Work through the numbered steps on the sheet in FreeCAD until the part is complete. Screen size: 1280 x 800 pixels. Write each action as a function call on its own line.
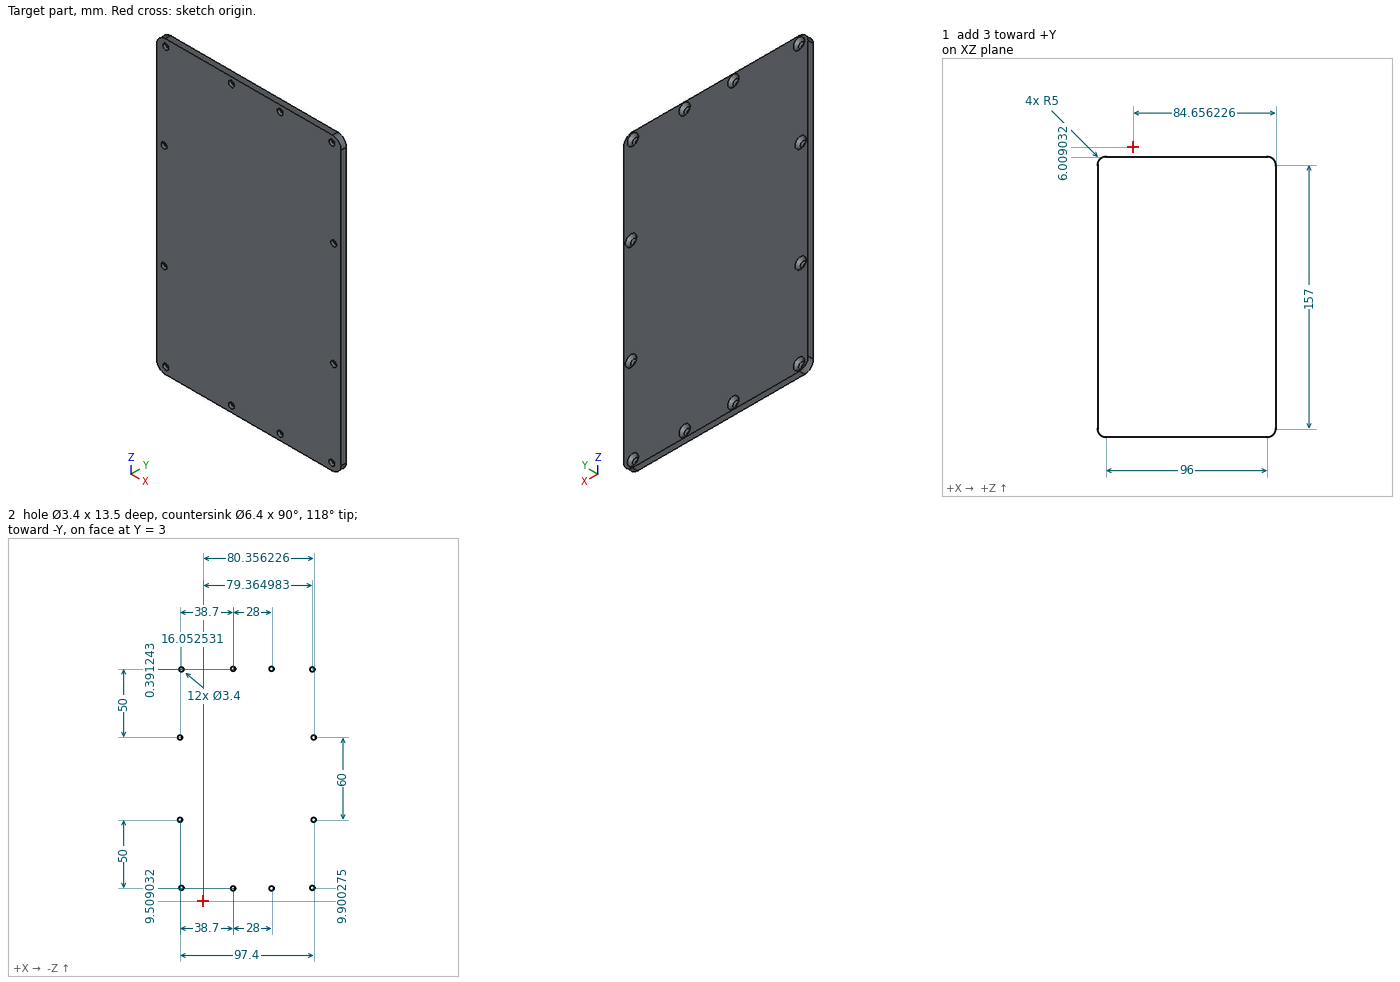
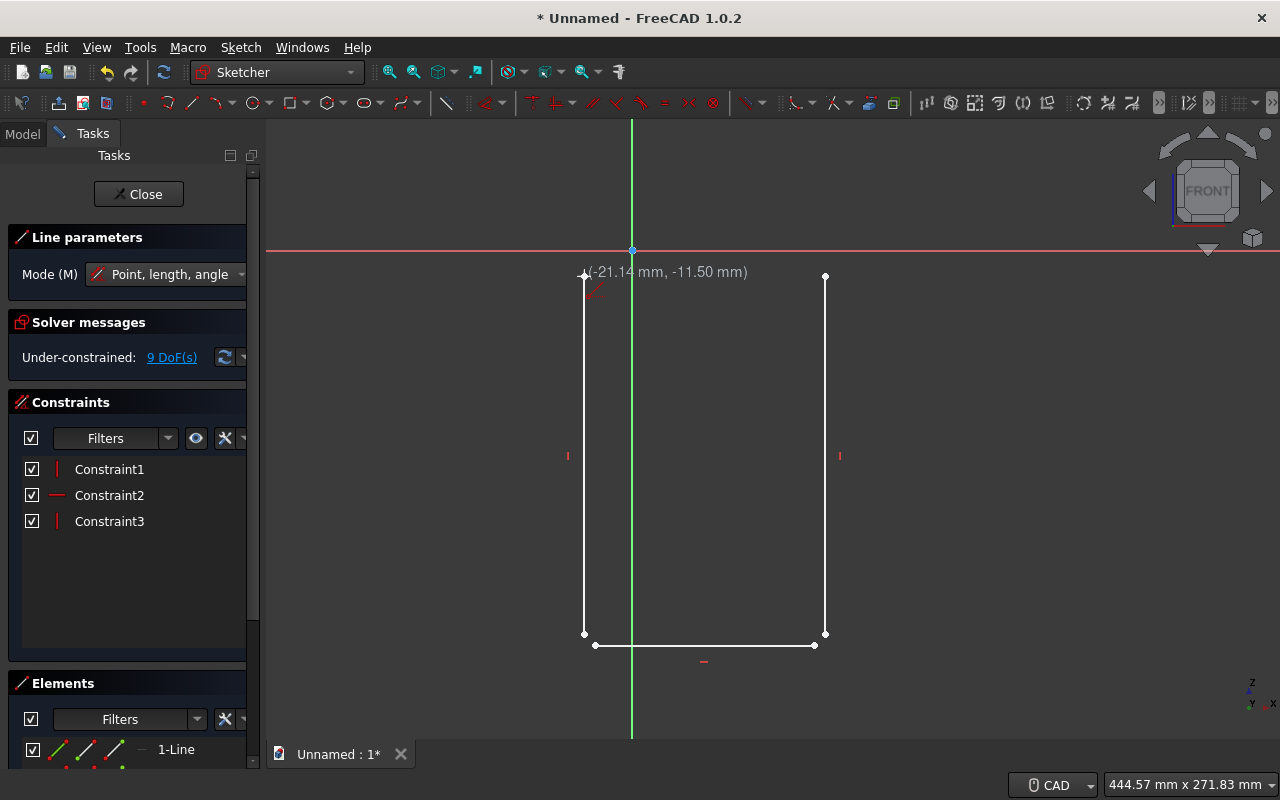
click(595, 264)
click(814, 264)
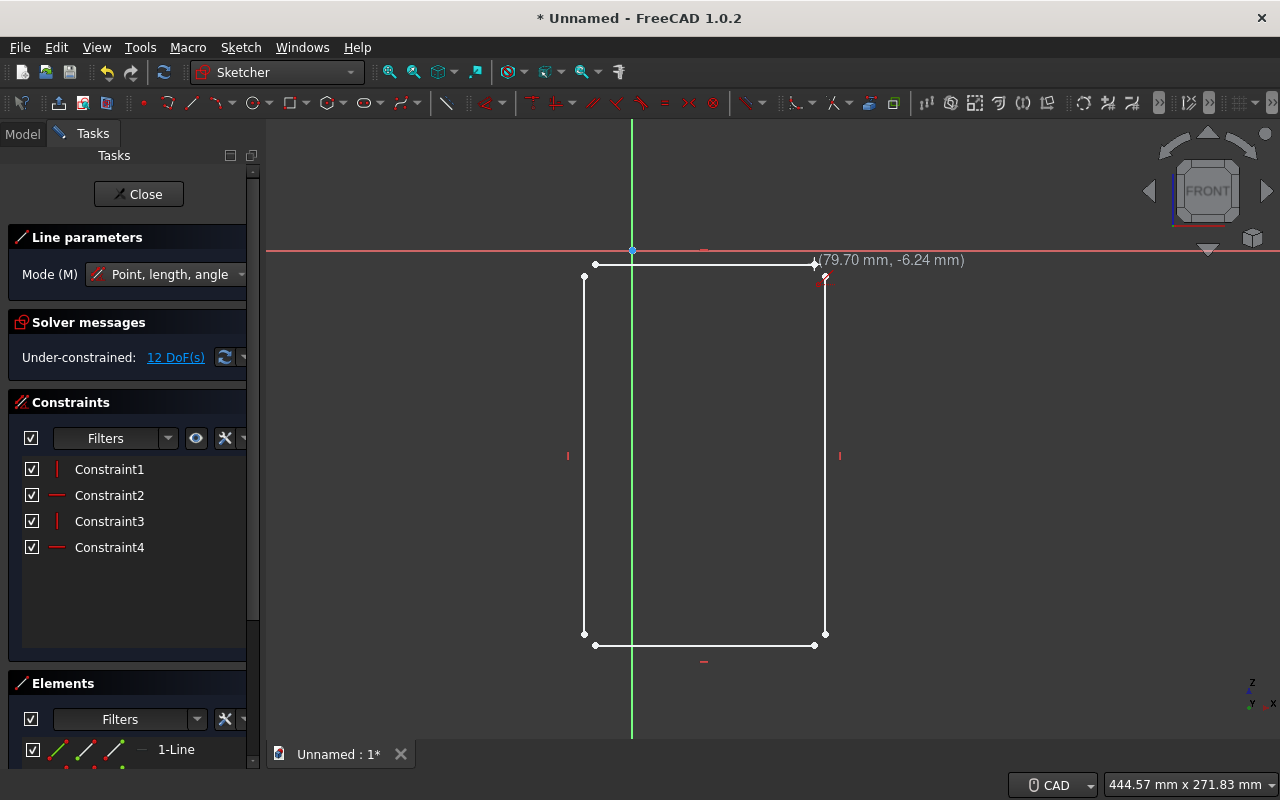
click(216, 104)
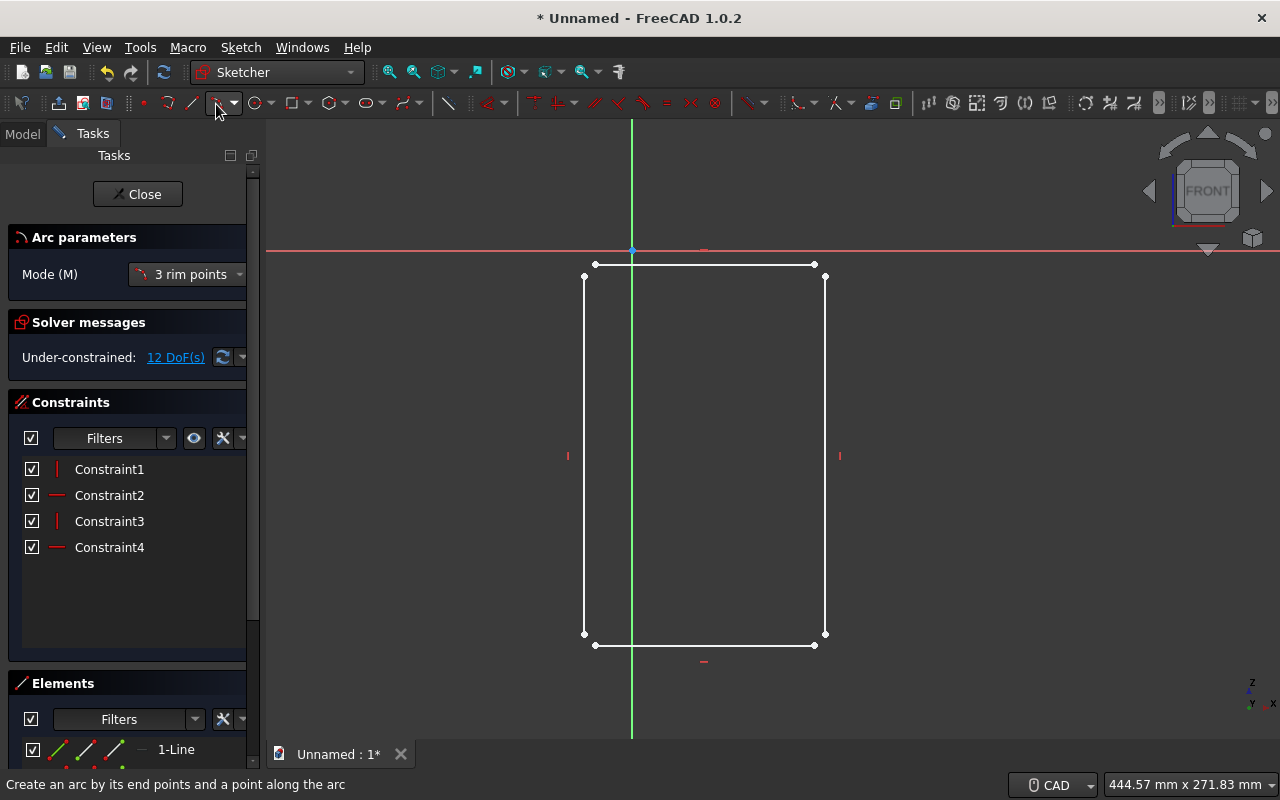
click(825, 635)
click(814, 646)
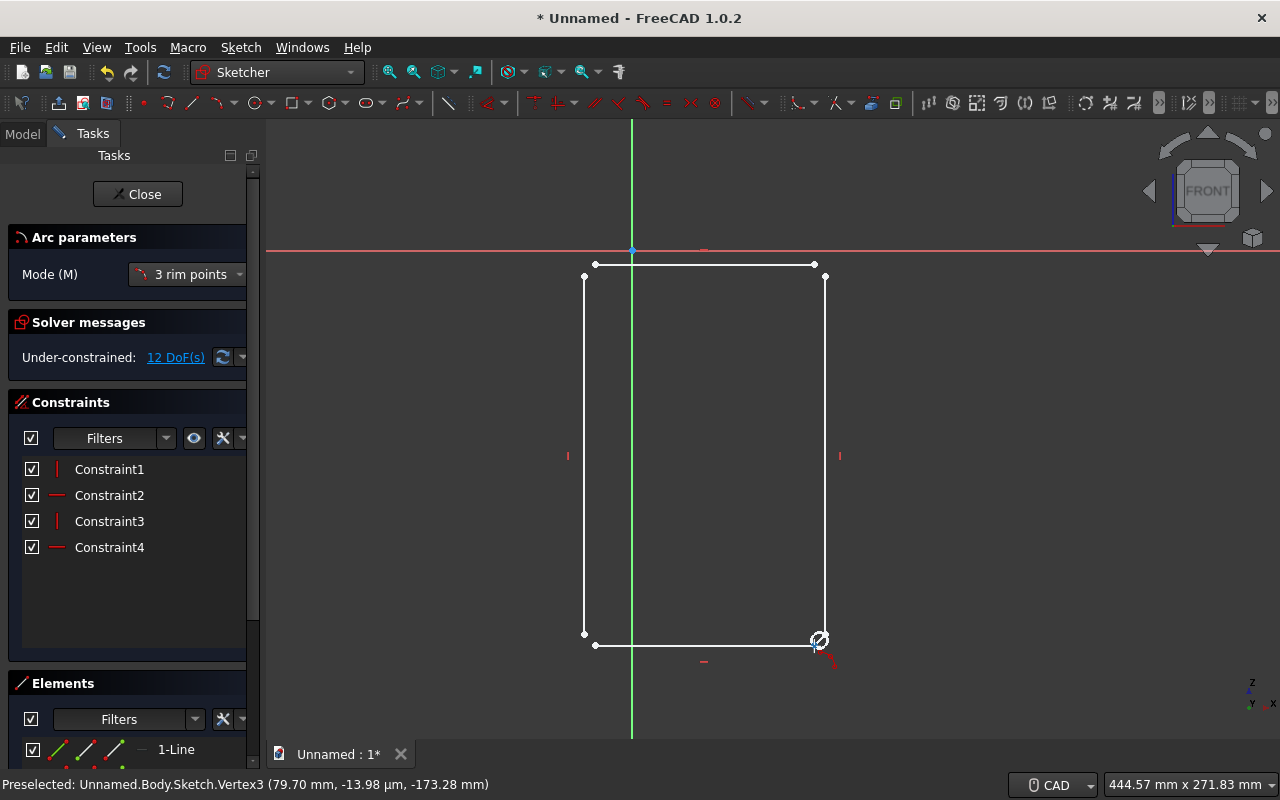
scroll(822, 642, up, 8)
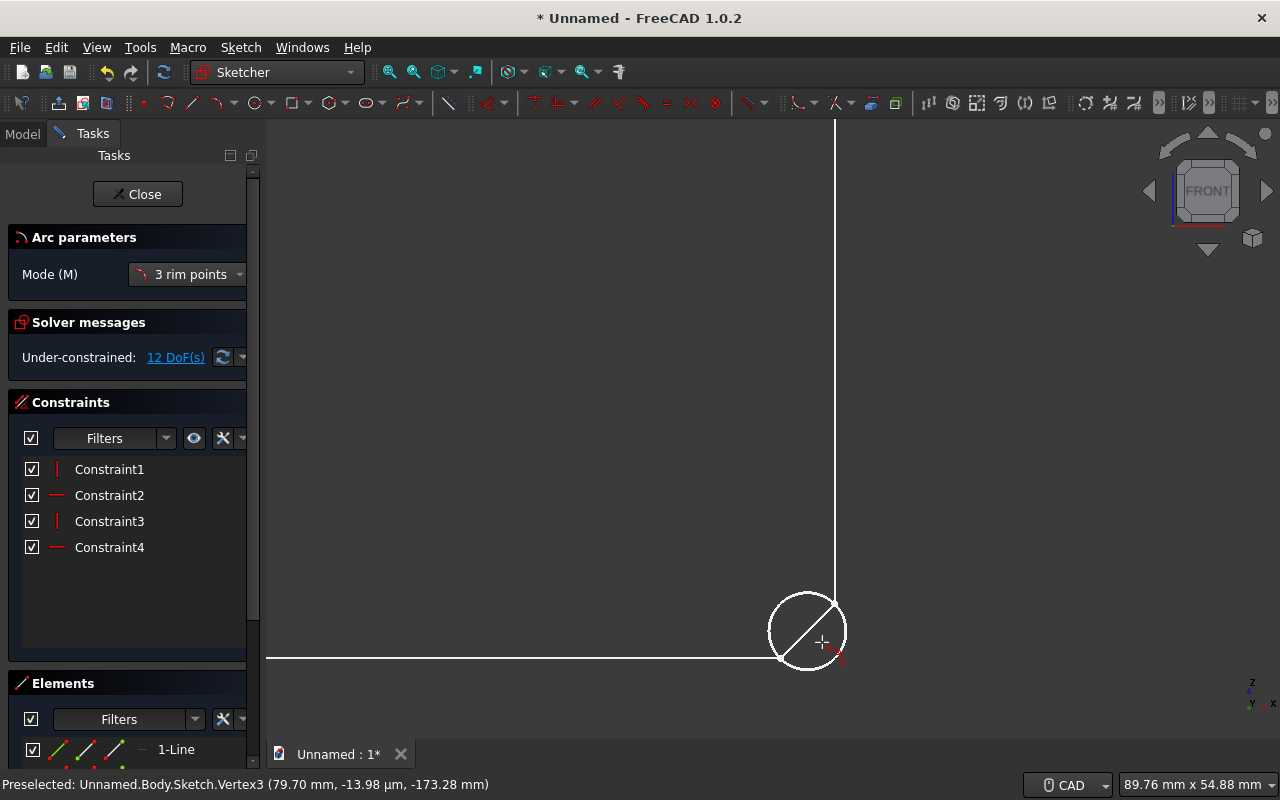
click(820, 639)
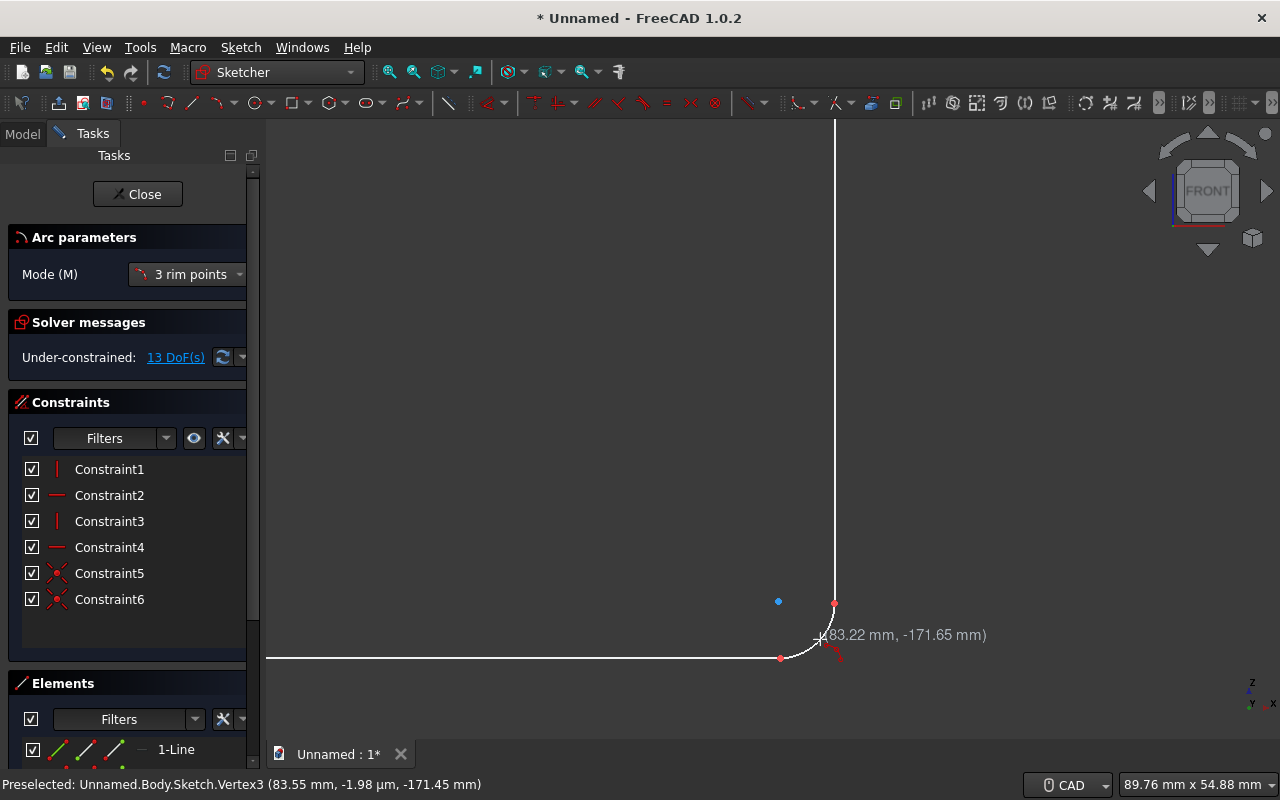
scroll(823, 619, down, 8)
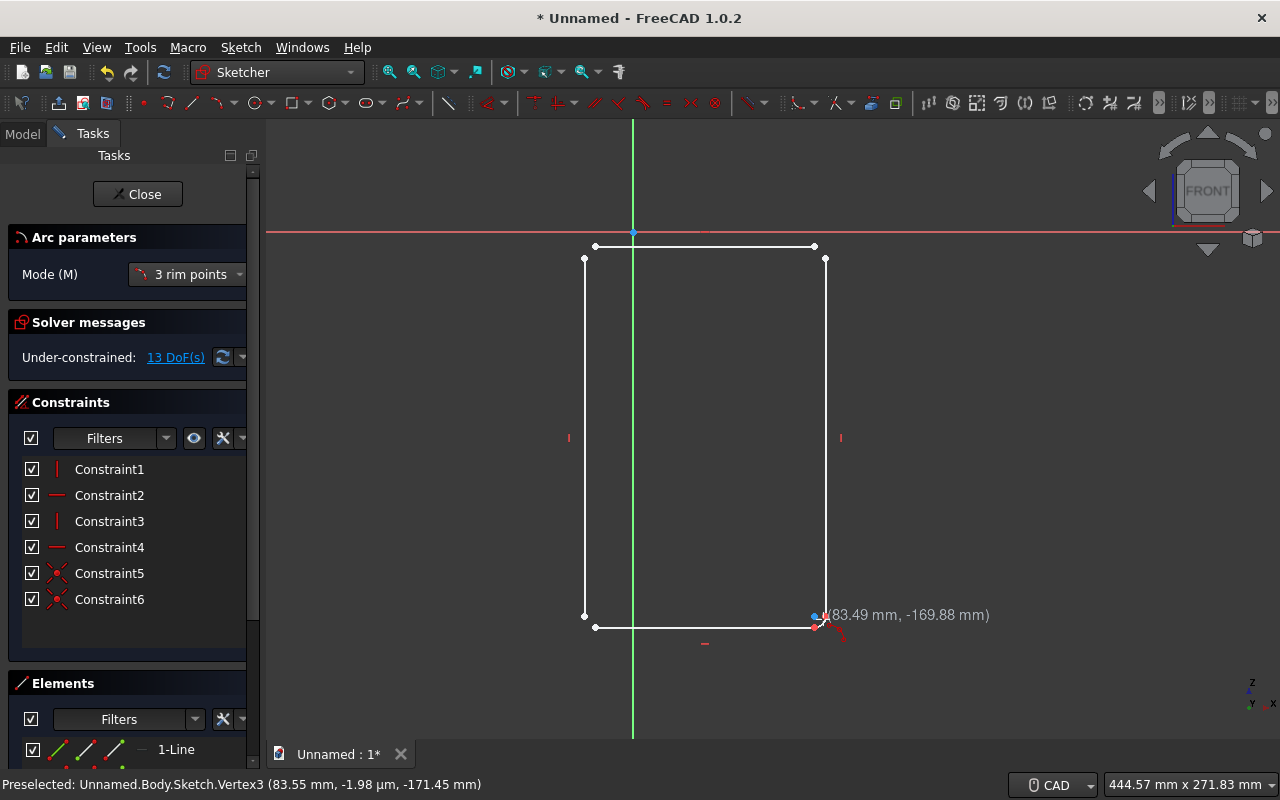
click(596, 628)
click(585, 617)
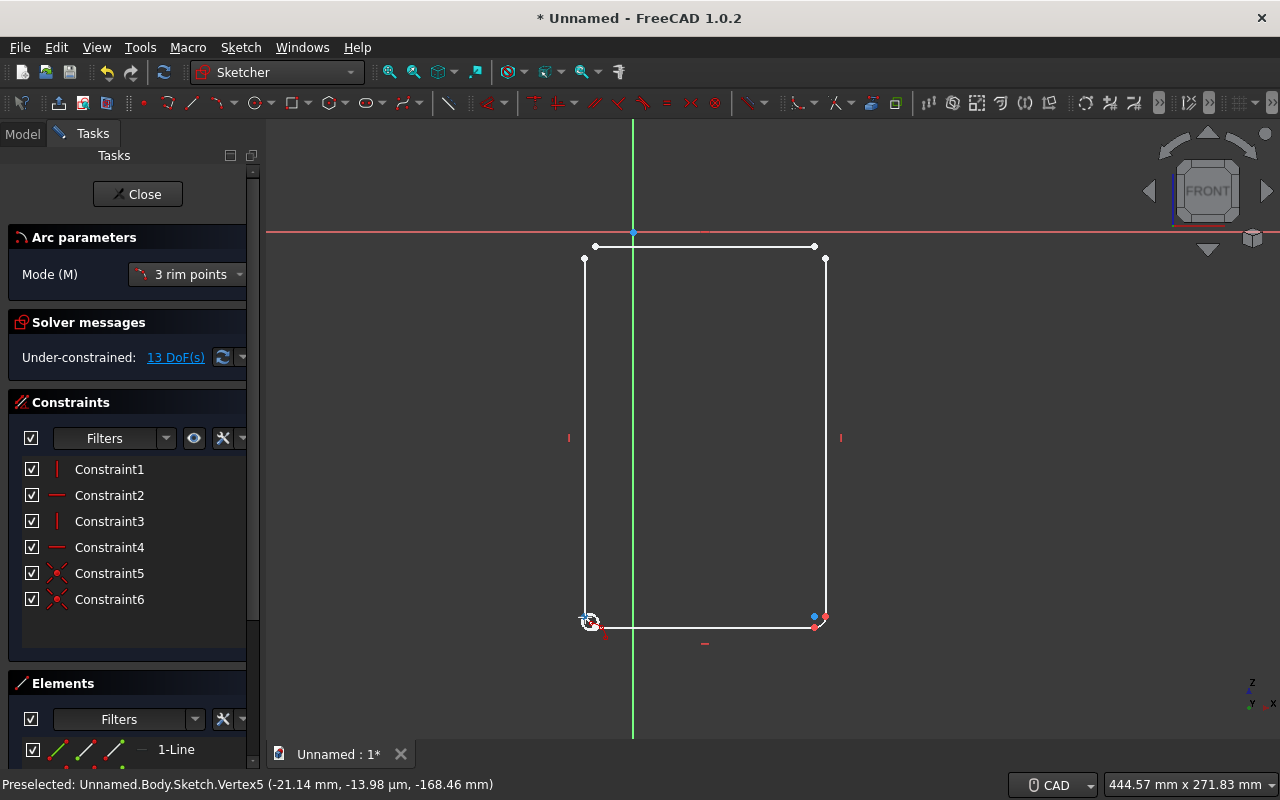
scroll(588, 624, up, 8)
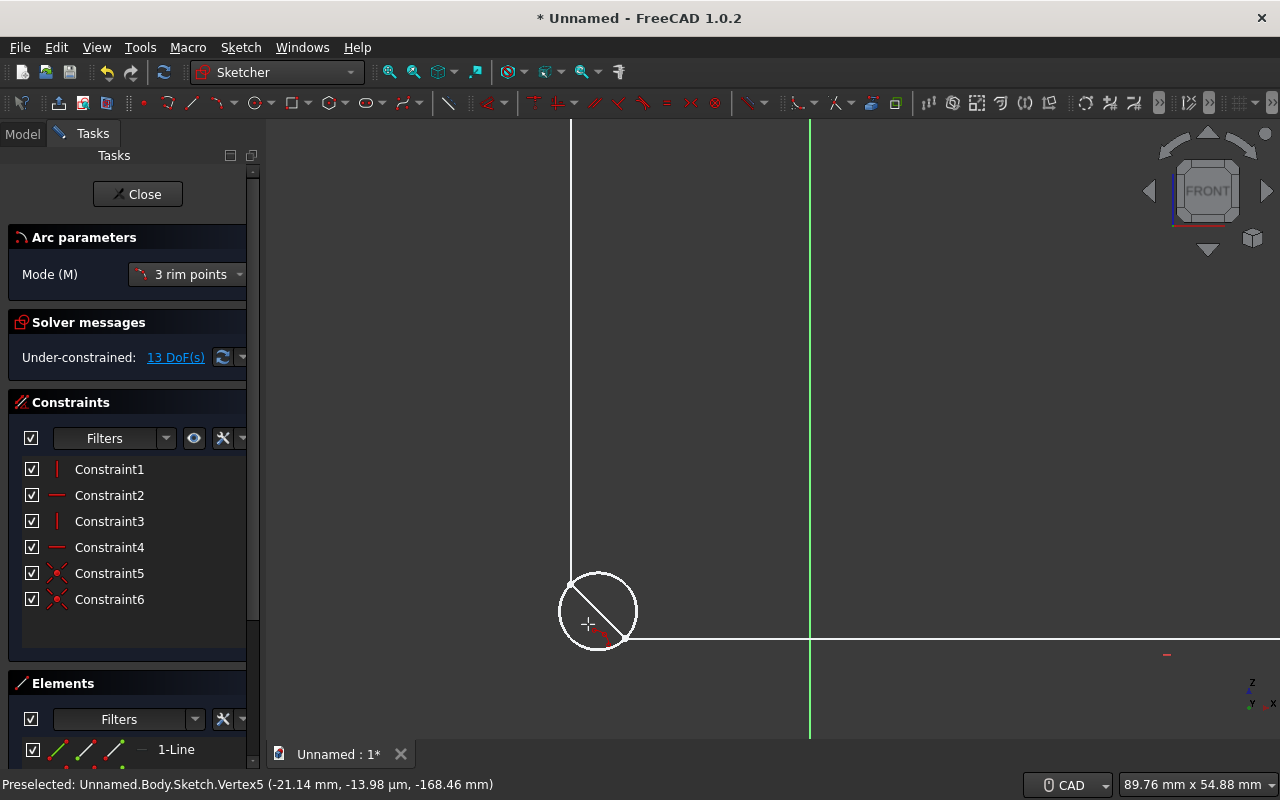
click(585, 619)